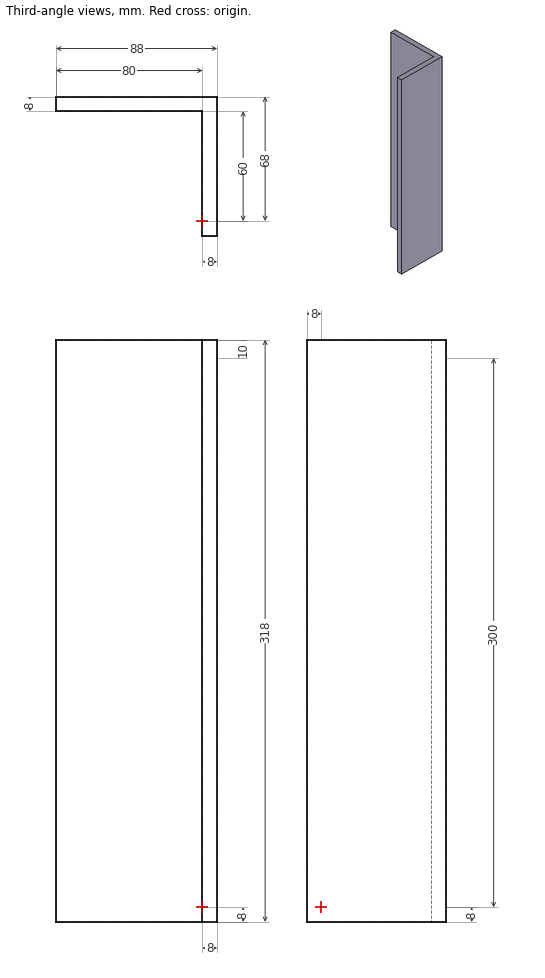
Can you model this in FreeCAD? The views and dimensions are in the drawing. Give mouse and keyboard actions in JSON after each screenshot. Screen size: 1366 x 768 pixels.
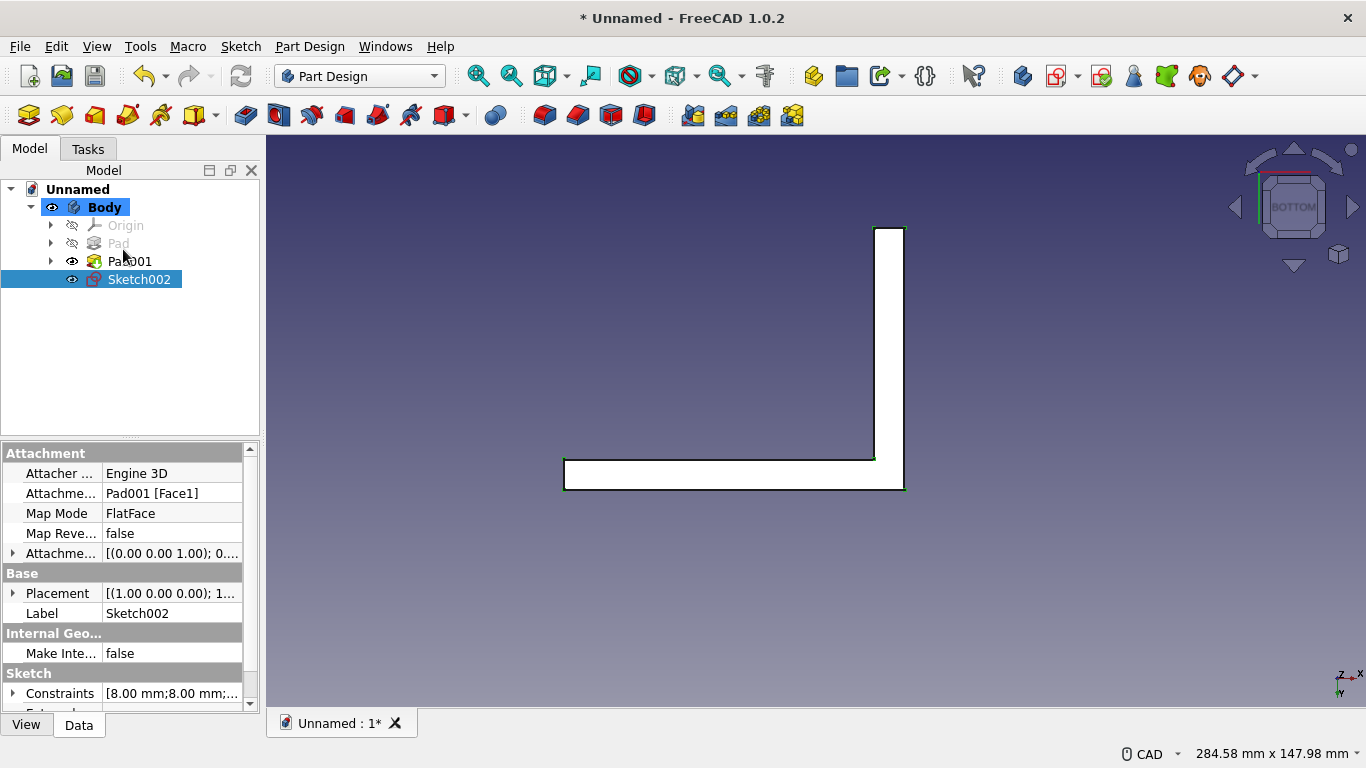
{"action": "left_click", "coordinate": [29, 116]}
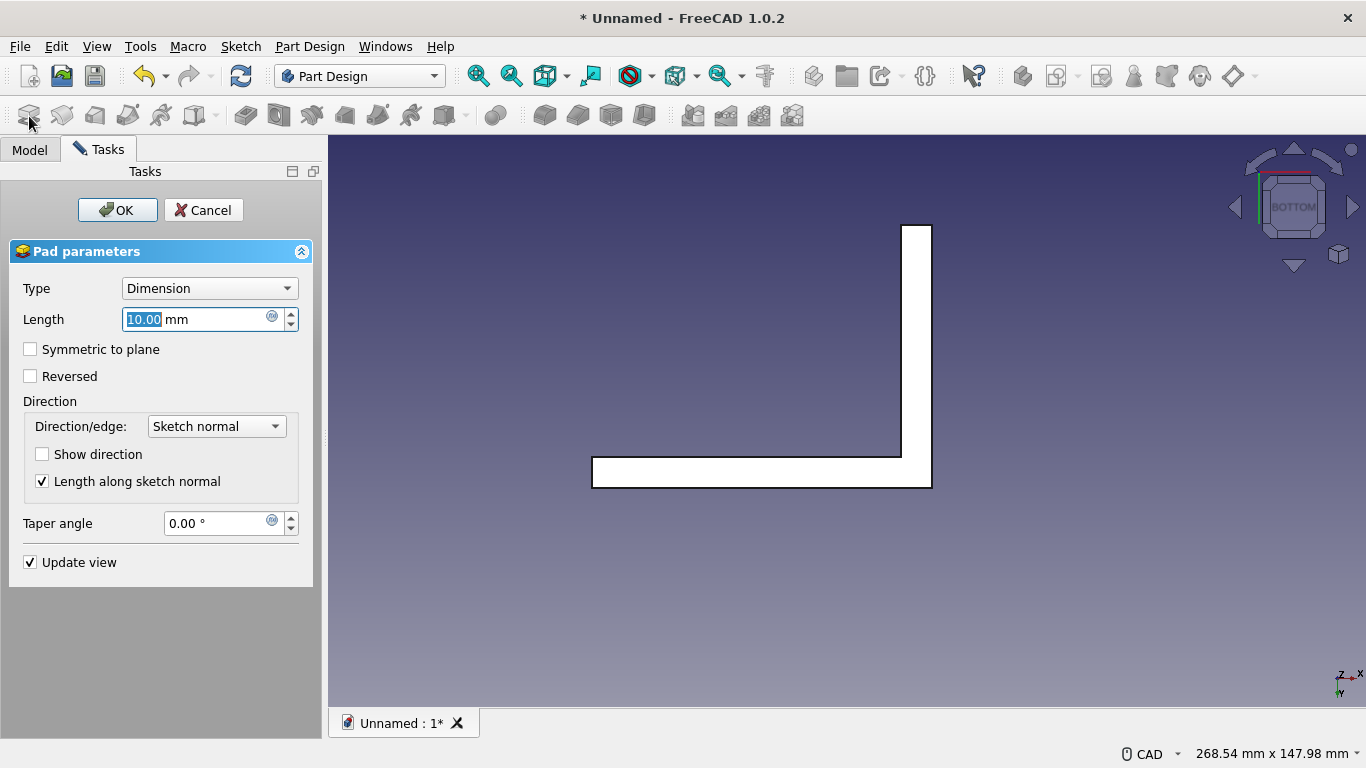
{"action": "type", "text": "8"}
{"action": "key", "text": "Tab"}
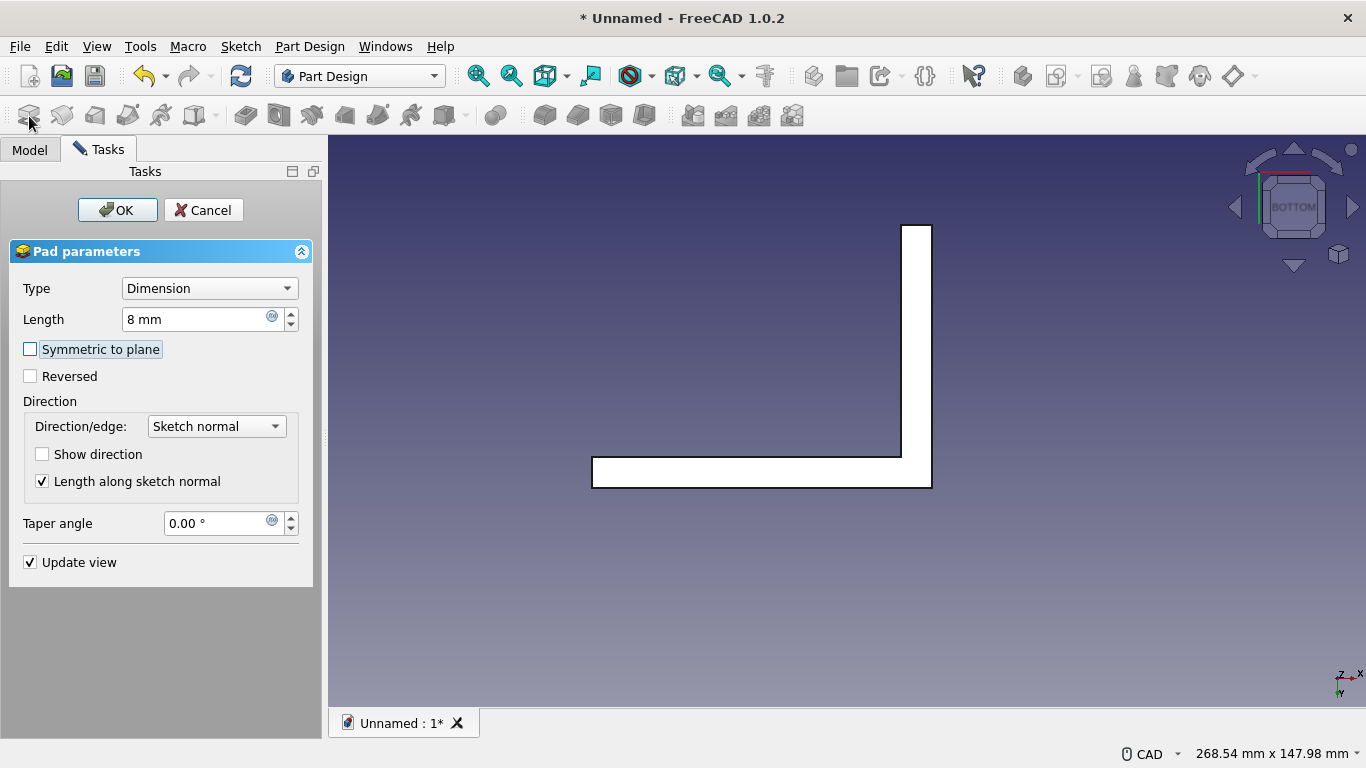
{"action": "left_click", "coordinate": [118, 210]}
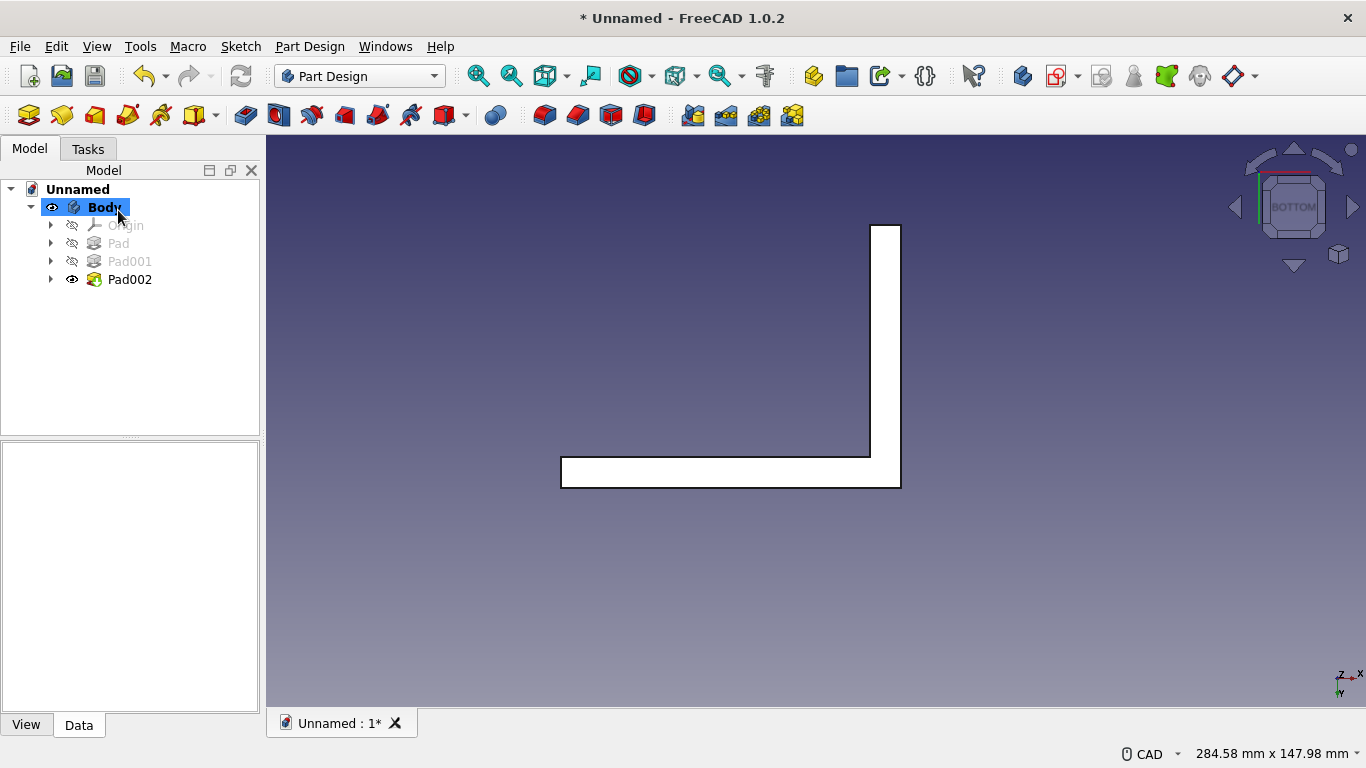
{"action": "key", "text": "0"}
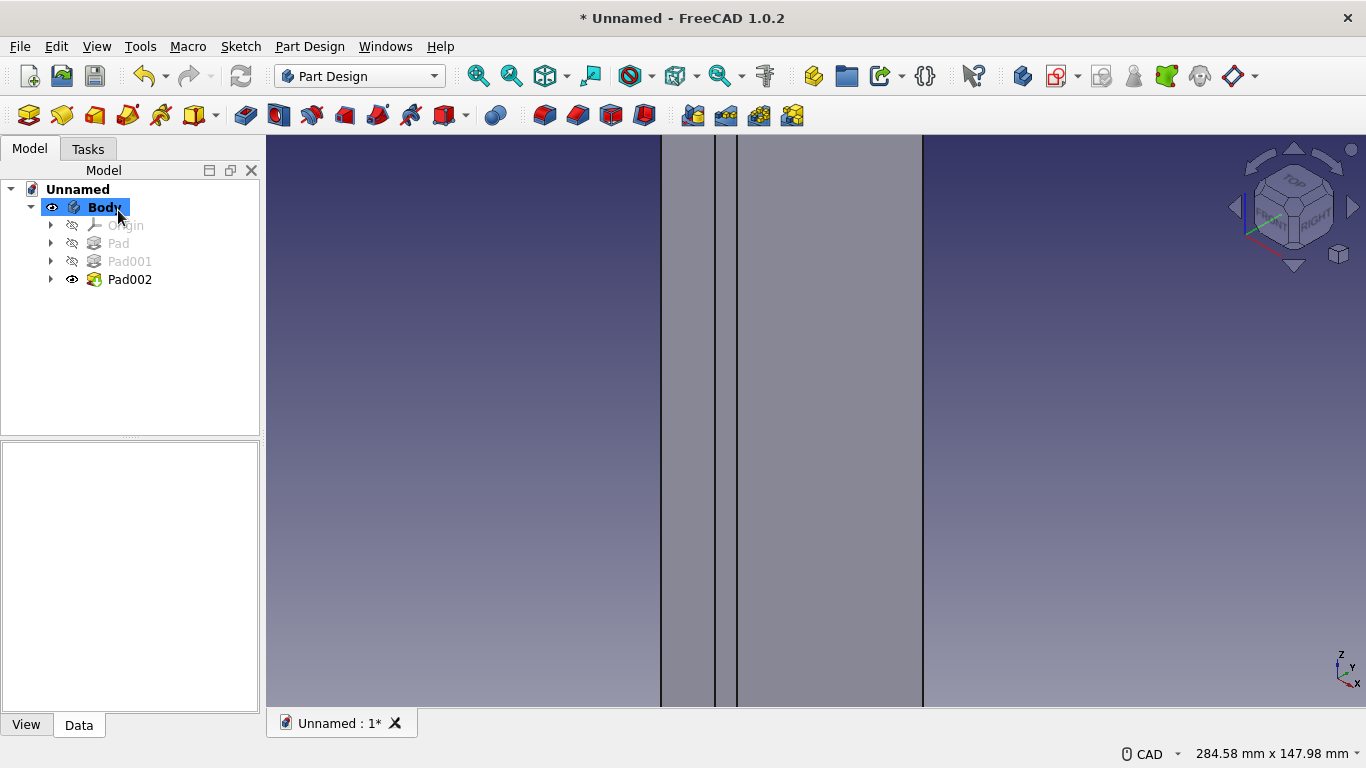
{"action": "left_click", "coordinate": [479, 76]}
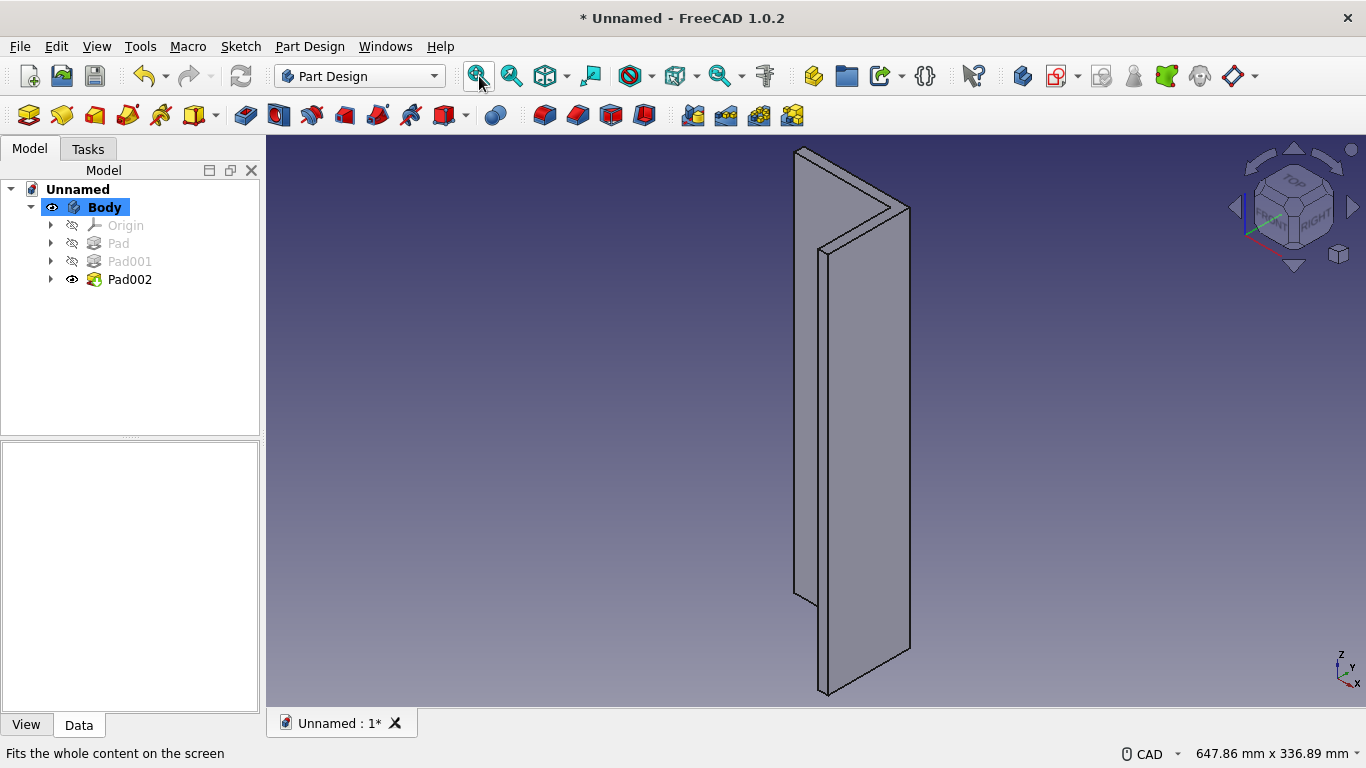
{"action": "scroll", "coordinate": [823, 282], "scroll_direction": "up", "scroll_amount": 3}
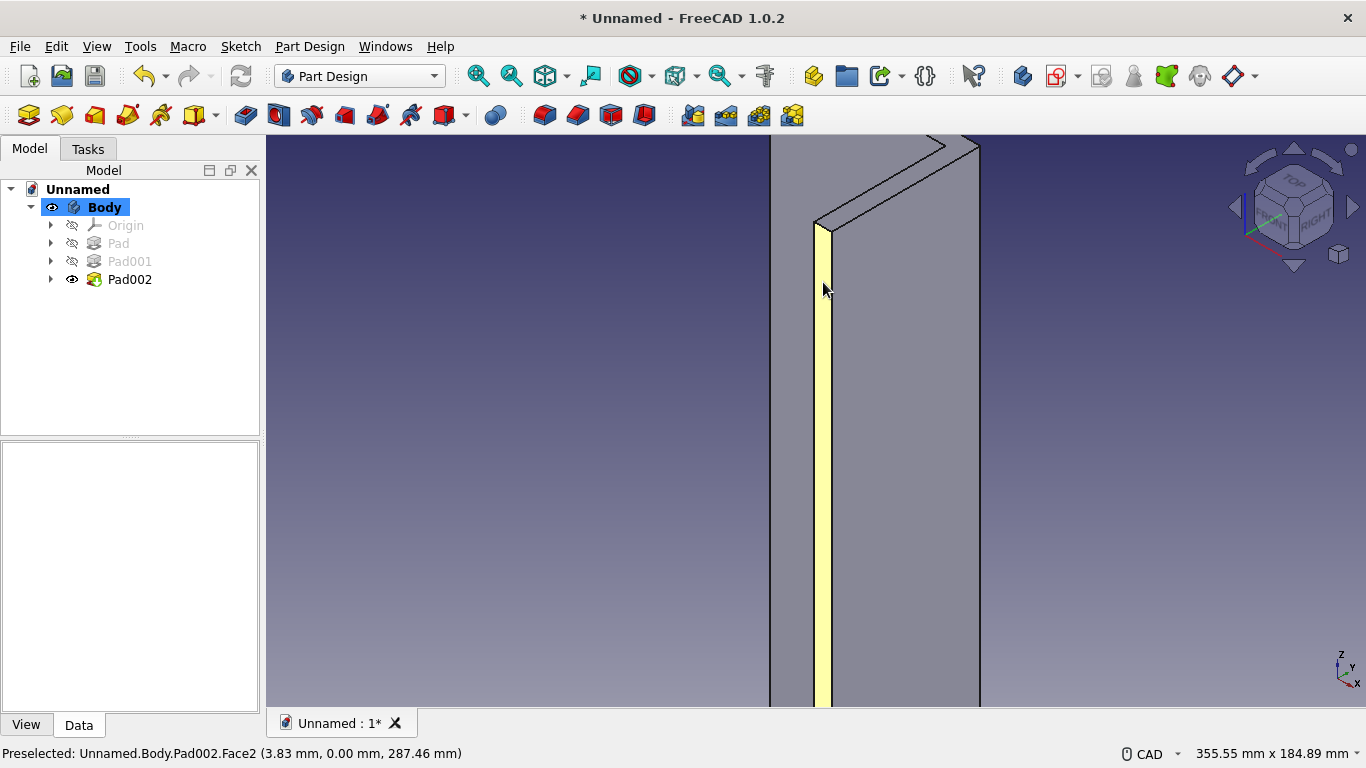
{"action": "left_click", "coordinate": [823, 283]}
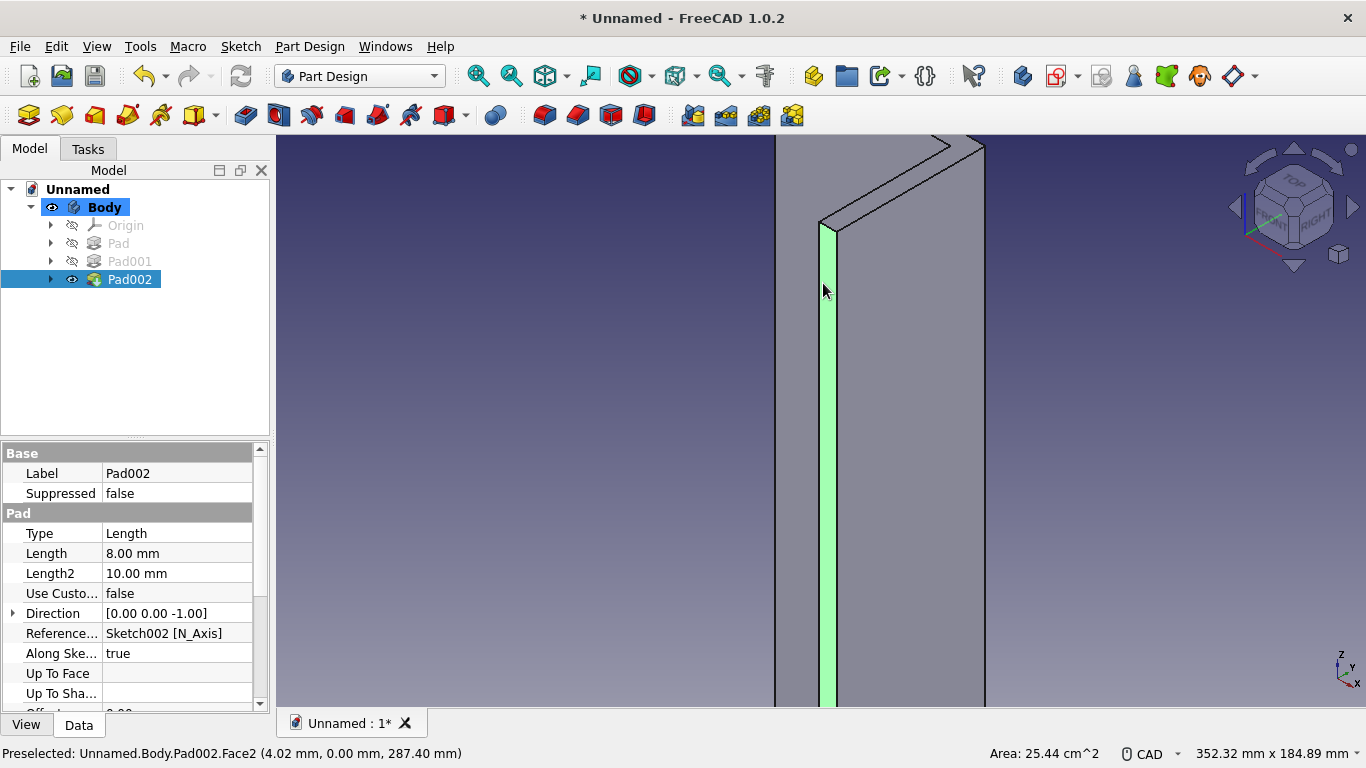
{"action": "left_click", "coordinate": [1056, 76]}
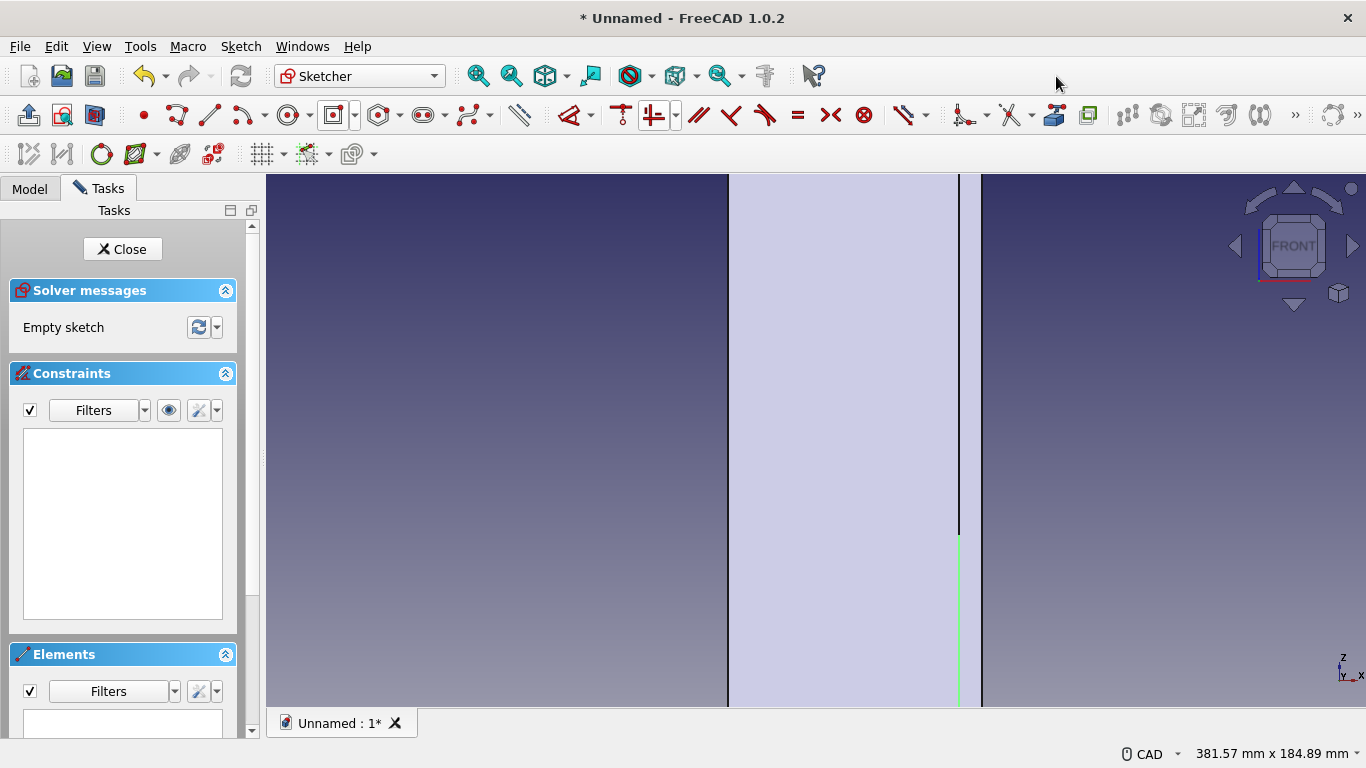
{"action": "scroll", "coordinate": [618, 390], "scroll_direction": "down", "scroll_amount": 5}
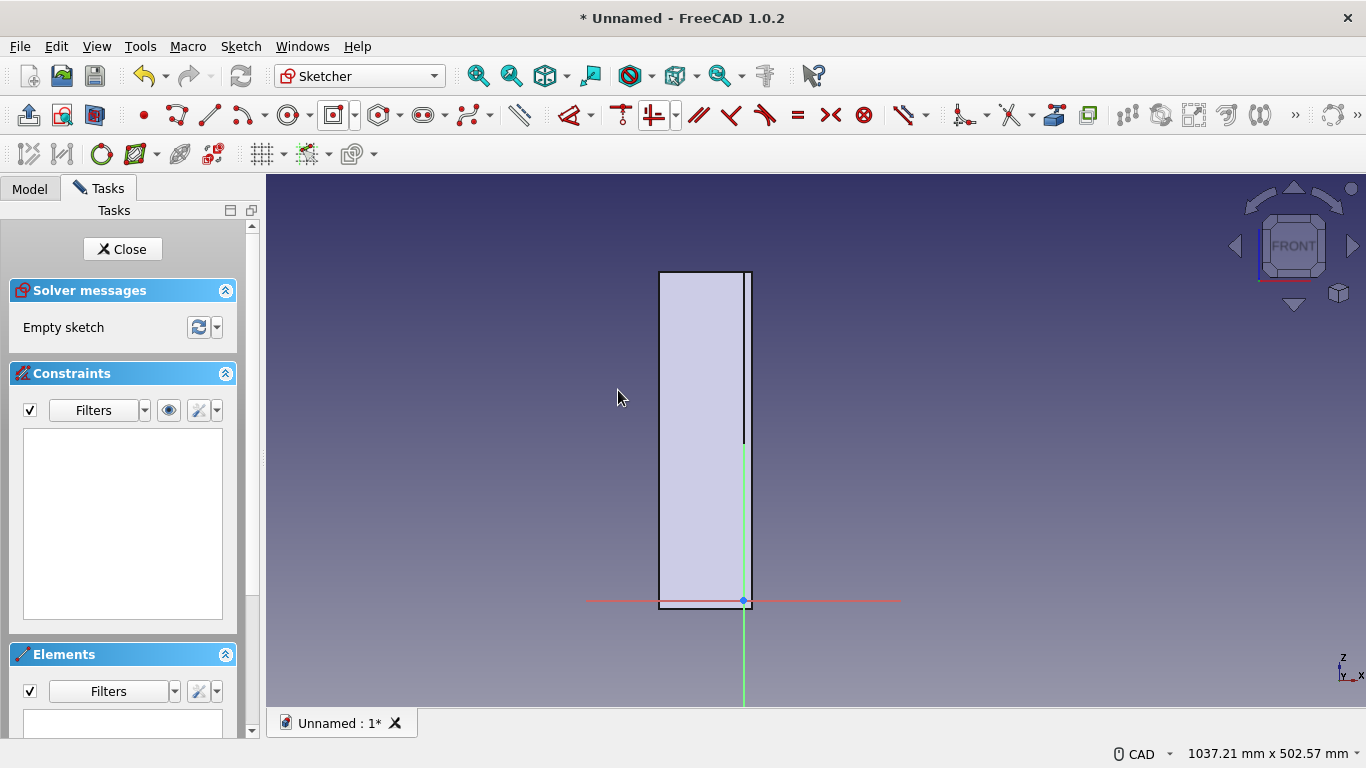
{"action": "left_click", "coordinate": [354, 116]}